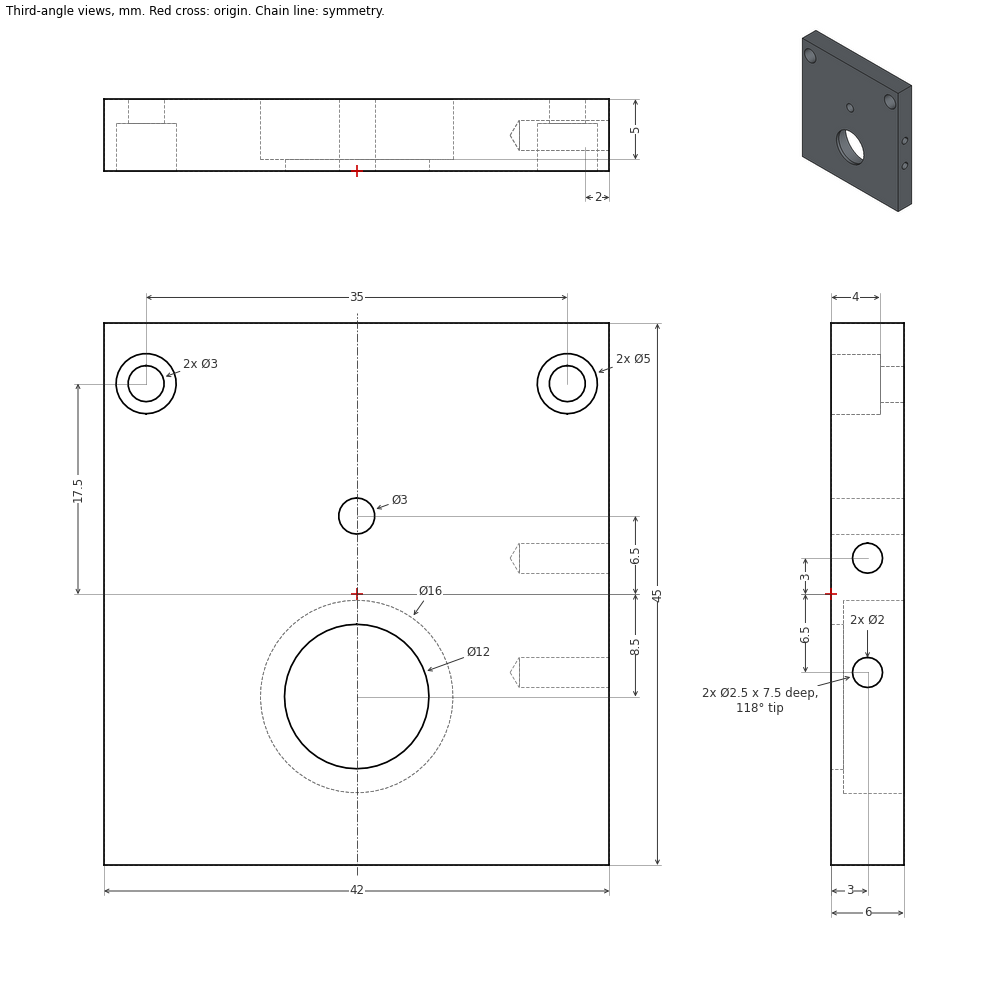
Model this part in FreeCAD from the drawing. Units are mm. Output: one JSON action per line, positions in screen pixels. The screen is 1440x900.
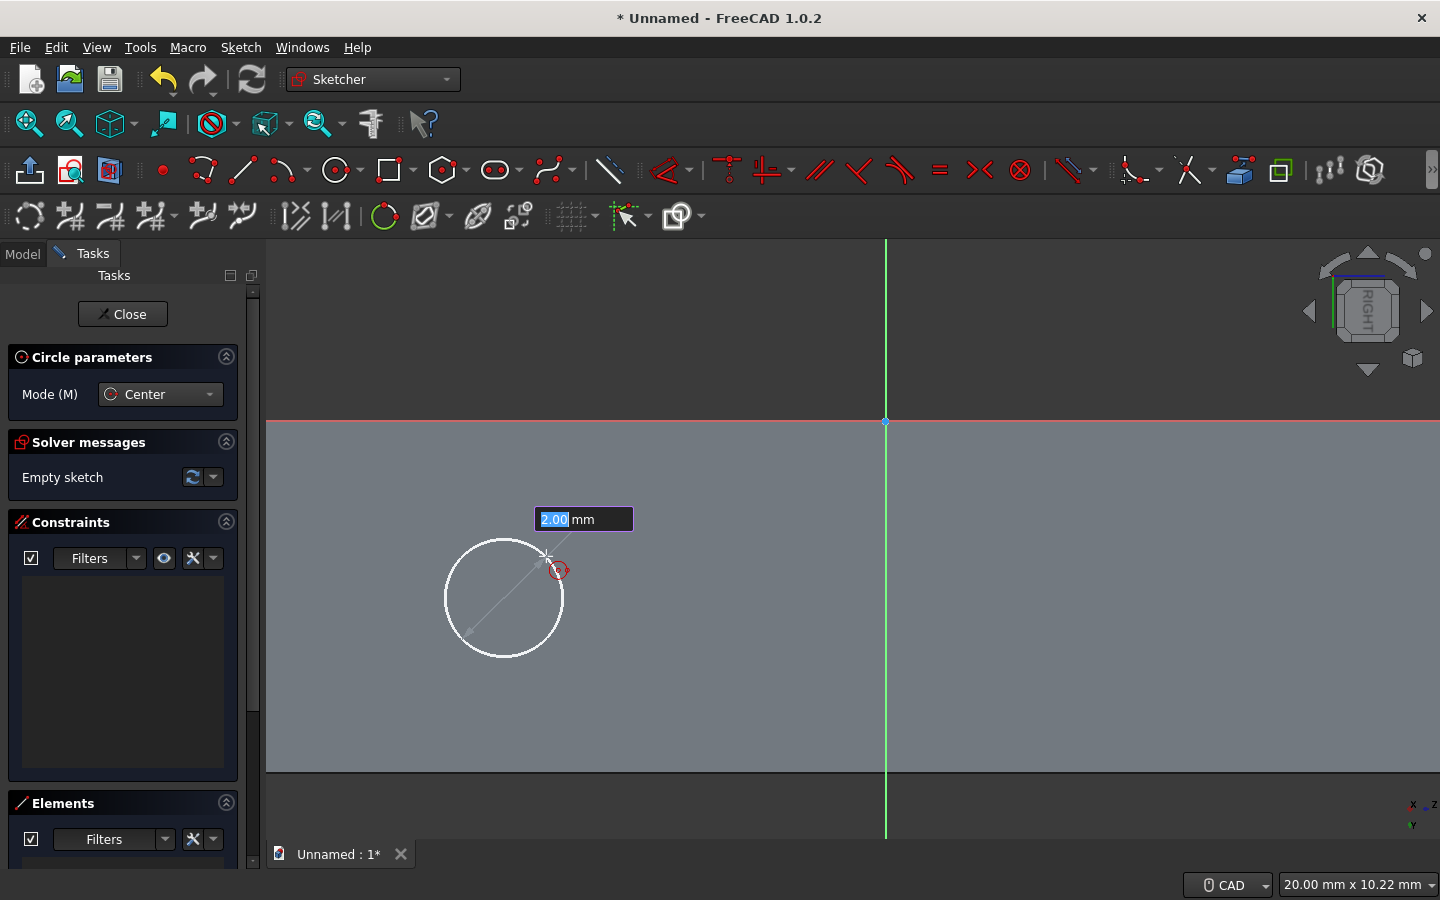
{"action": "type", "text": "2"}
{"action": "key", "text": "Return"}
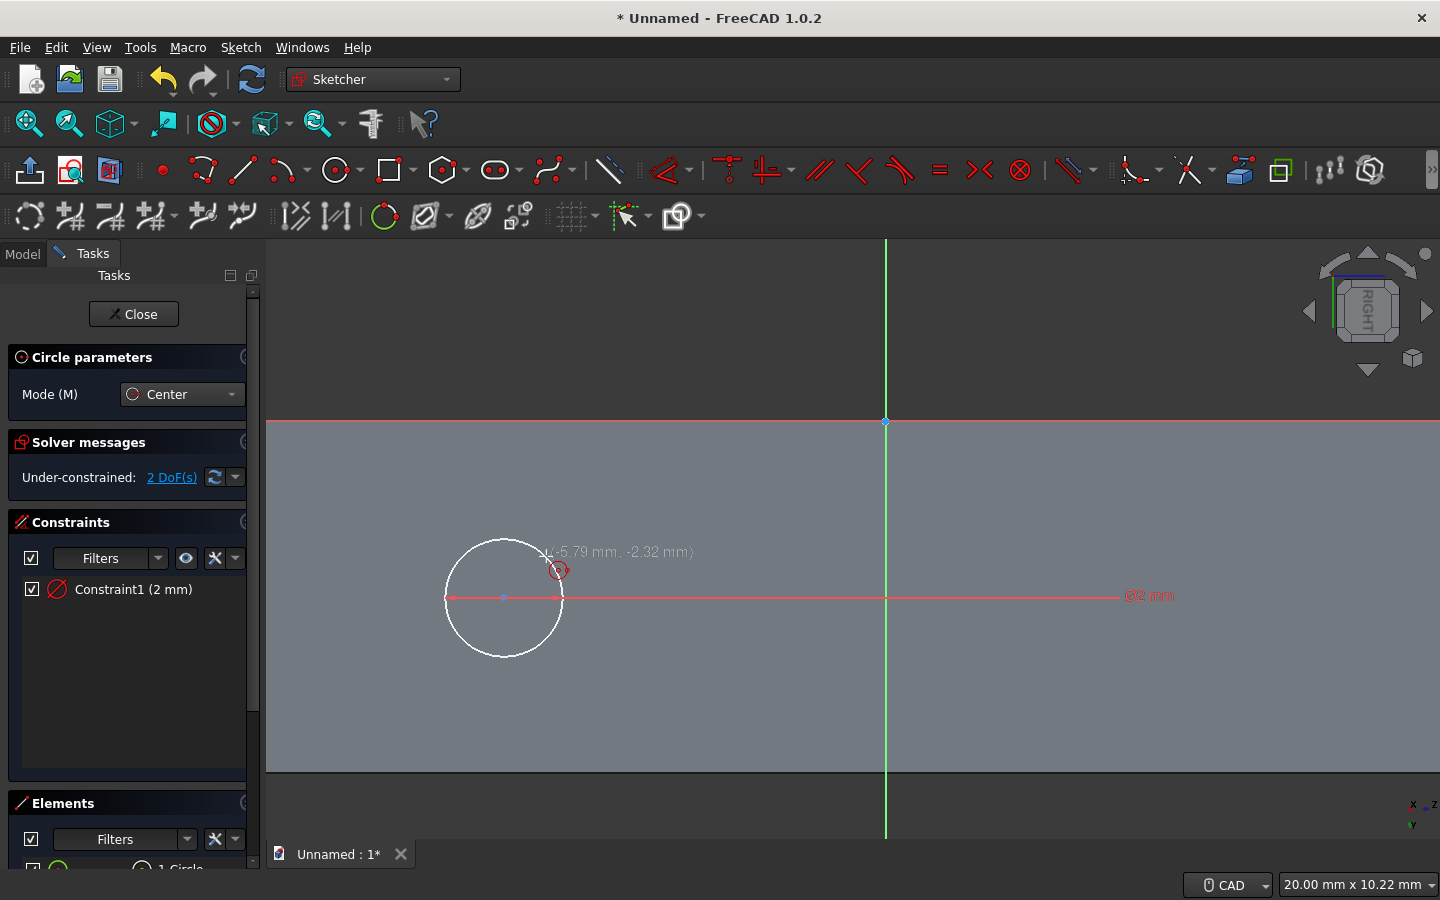
{"action": "left_click", "coordinate": [1062, 597]}
{"action": "mouse_move", "coordinate": [1103, 556]}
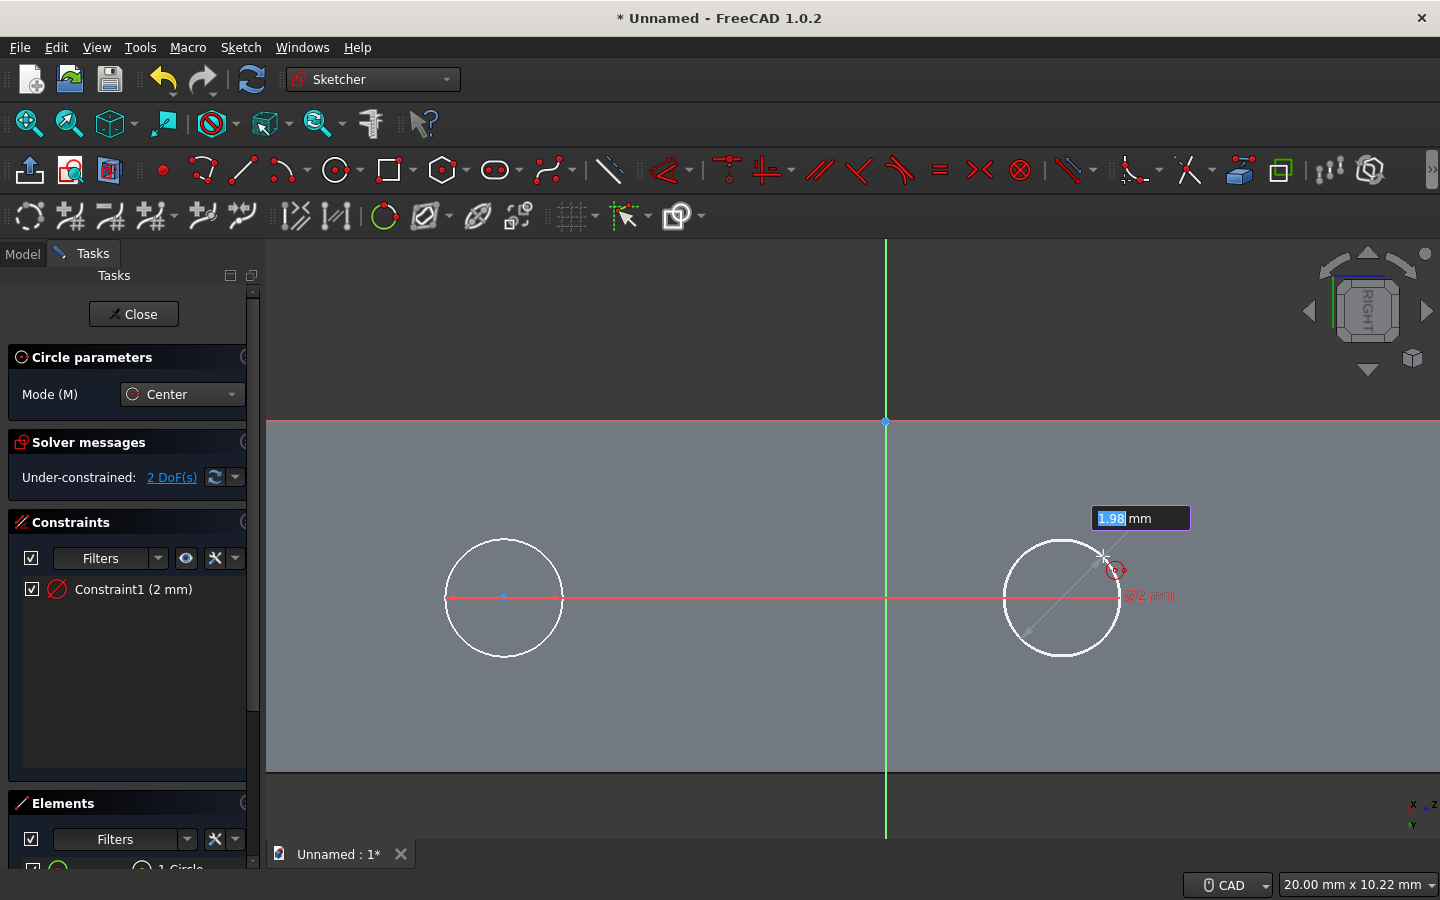
{"action": "type", "text": "2"}
{"action": "key", "text": "Return"}
{"action": "key", "text": "Escape"}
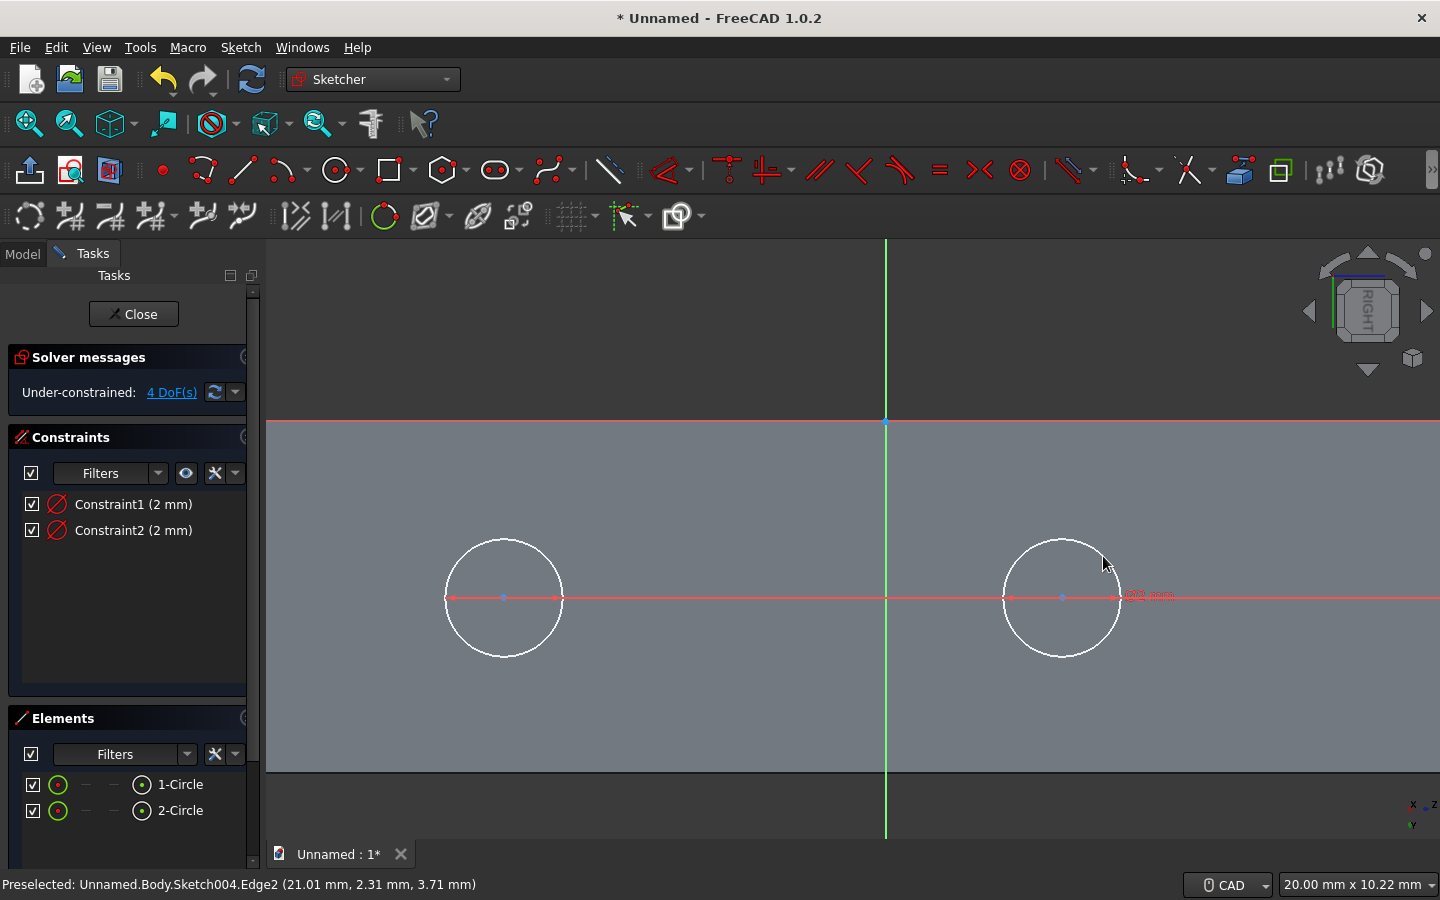
{"action": "left_click", "coordinate": [664, 170]}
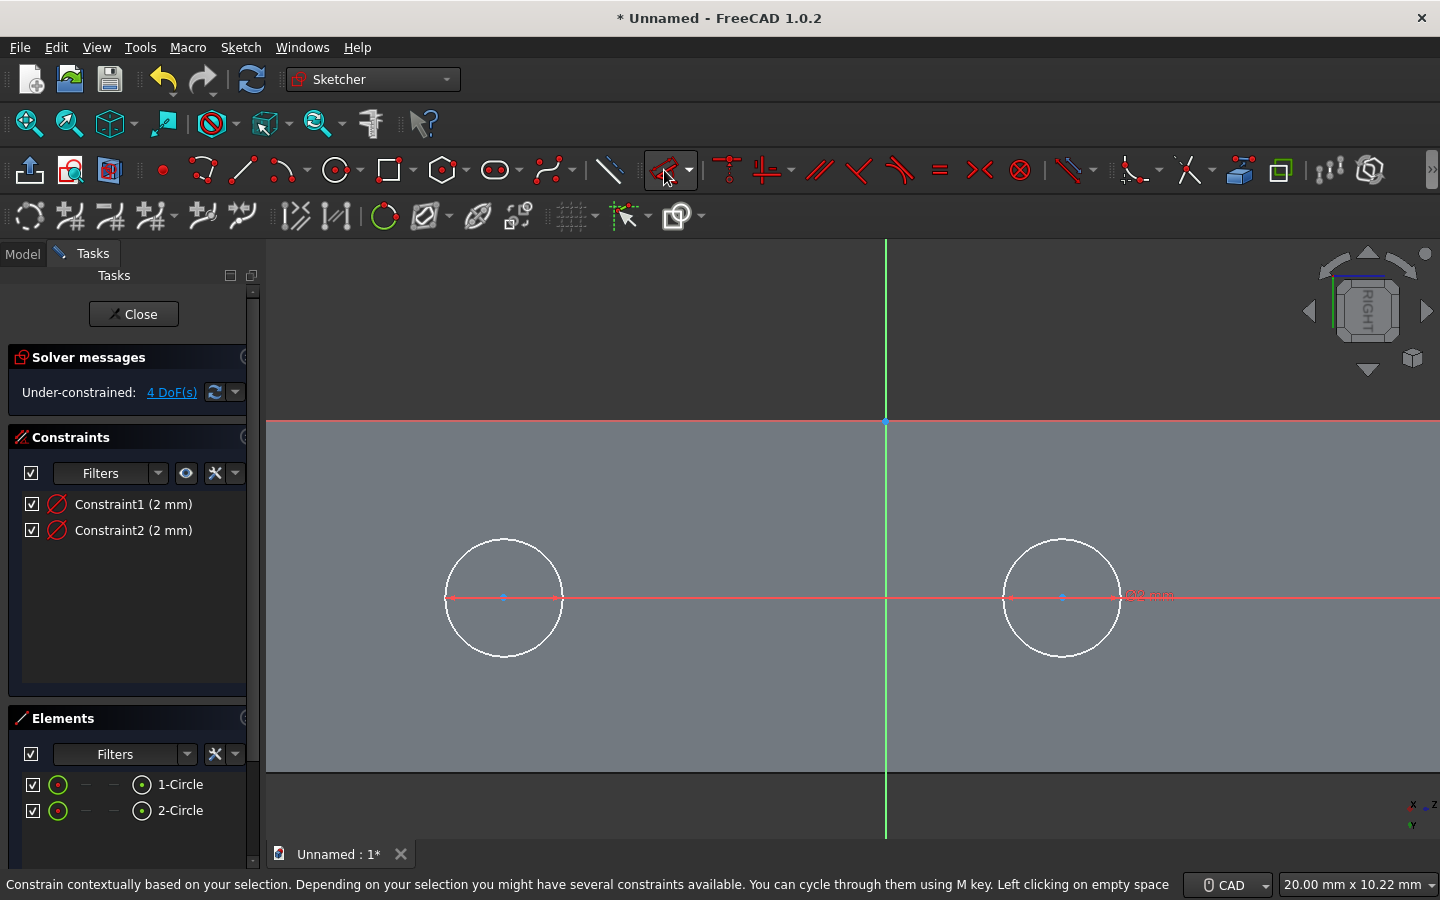
{"action": "left_click", "coordinate": [504, 598]}
{"action": "left_click", "coordinate": [470, 510]}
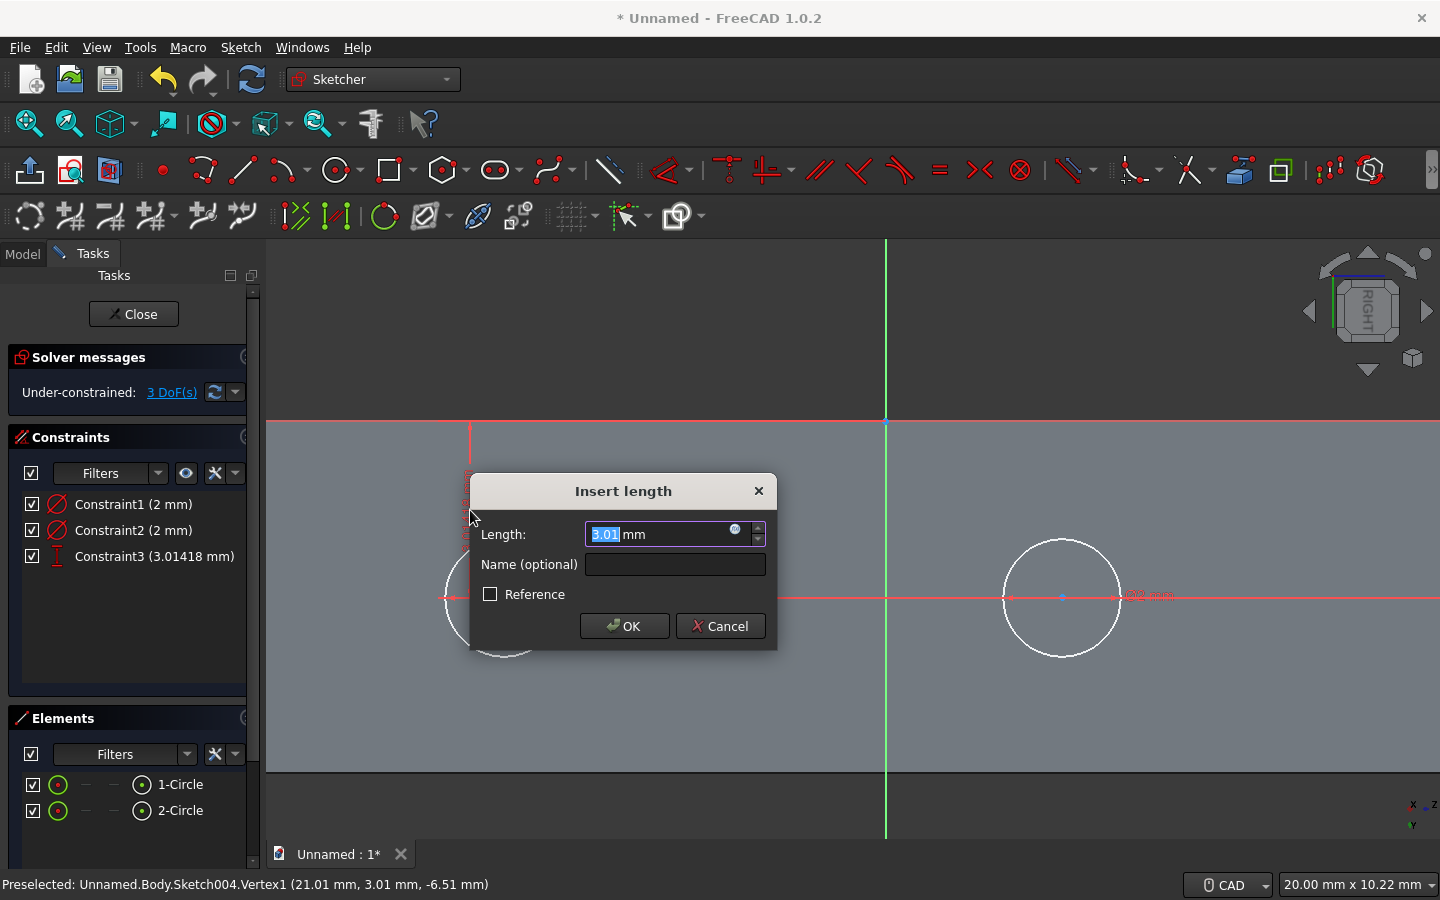
{"action": "type", "text": "3"}
{"action": "key", "text": "Return"}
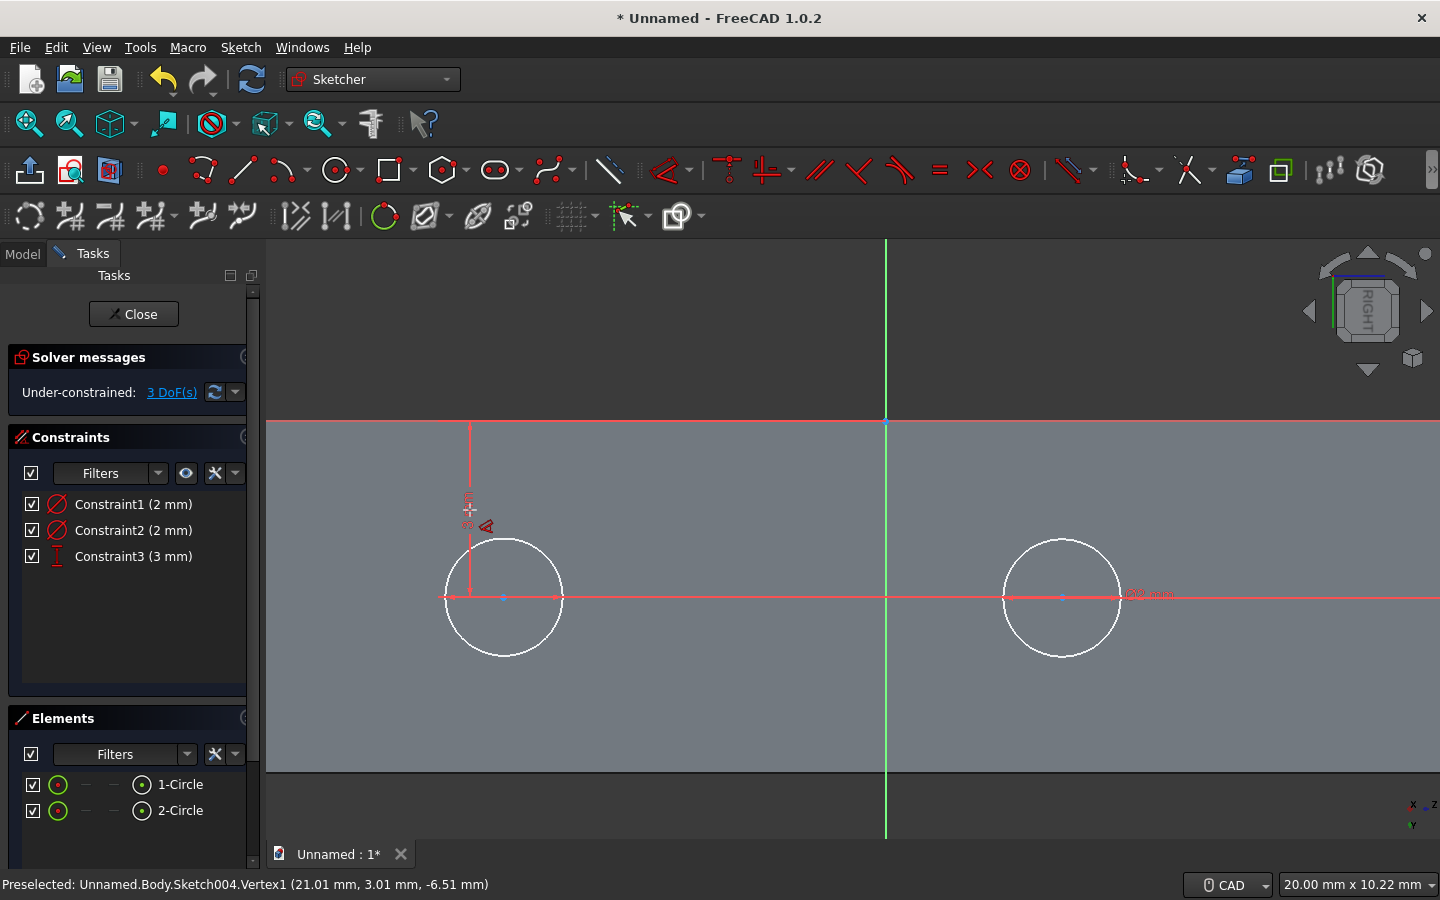
{"action": "left_click", "coordinate": [1062, 598]}
{"action": "left_click", "coordinate": [974, 387]}